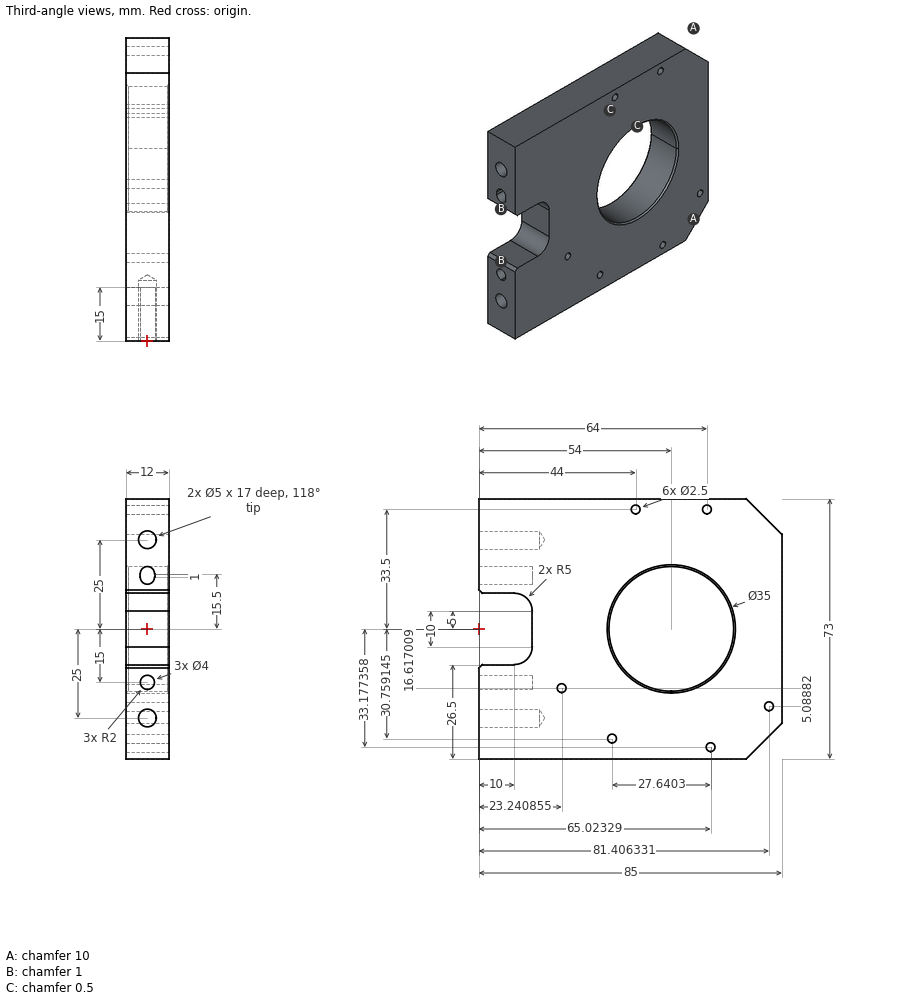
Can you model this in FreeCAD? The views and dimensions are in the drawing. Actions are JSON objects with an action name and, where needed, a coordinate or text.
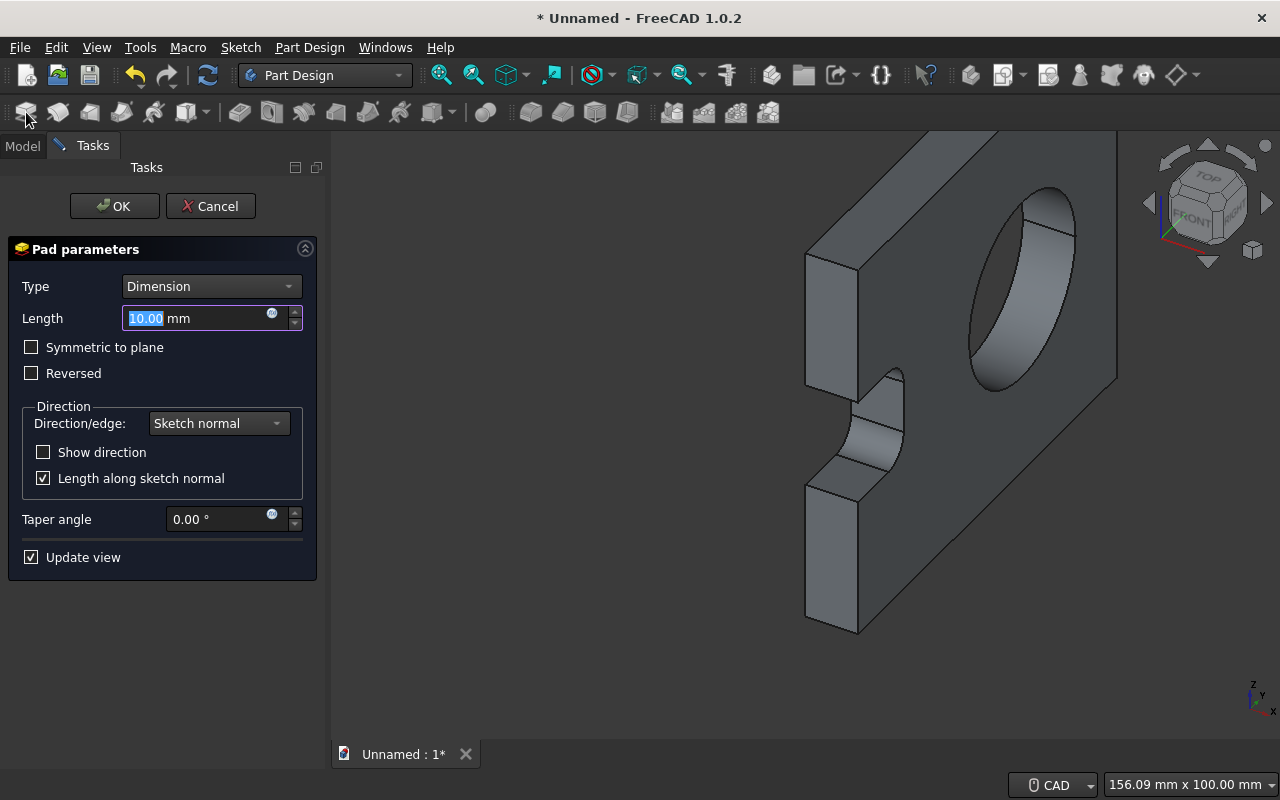
{"action": "type", "text": "12"}
{"action": "key", "text": "Tab"}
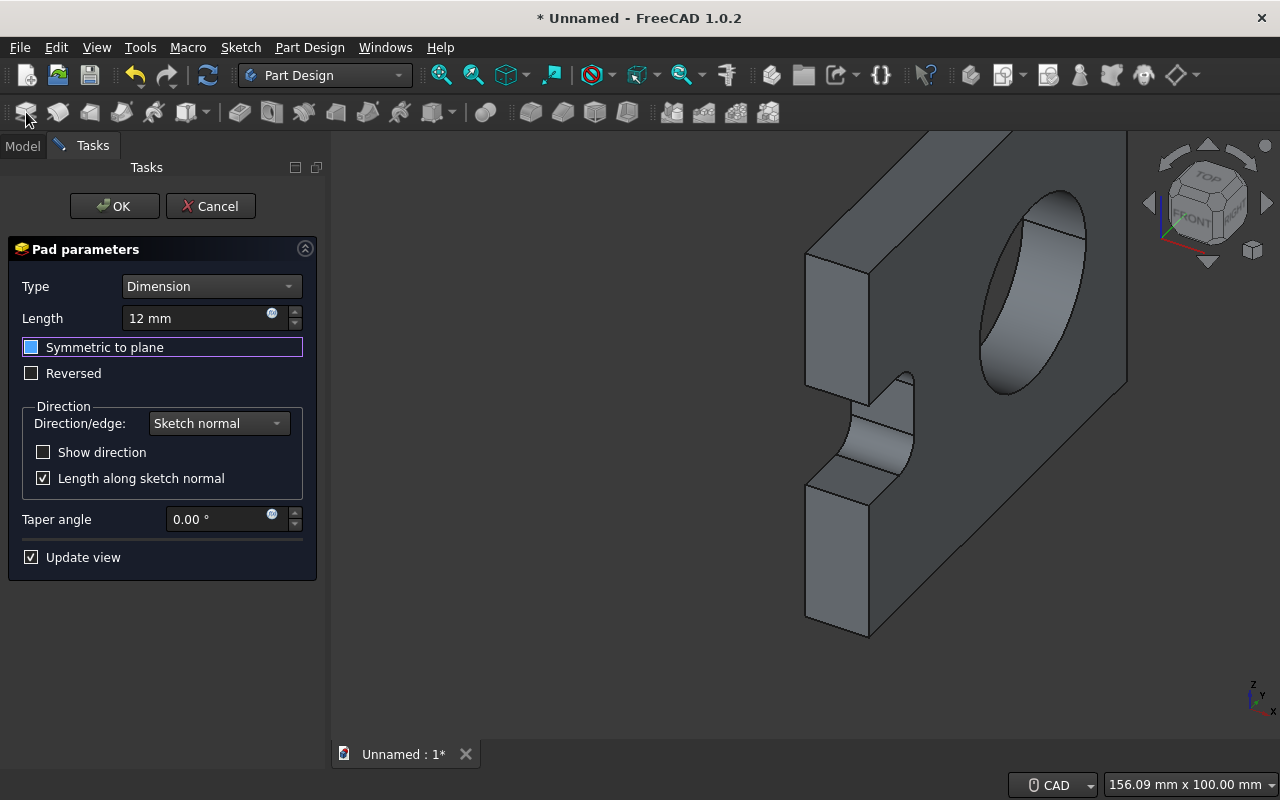
{"action": "left_click", "coordinate": [30, 347]}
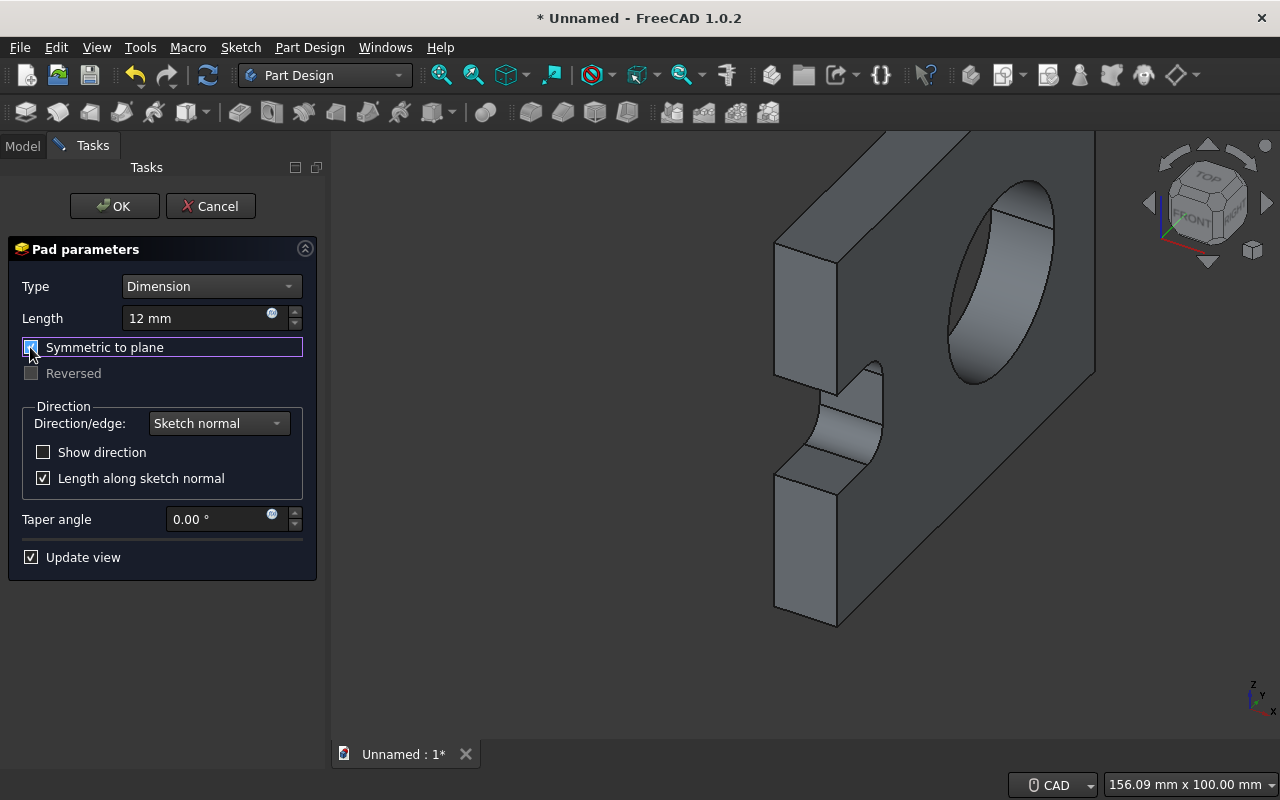
{"action": "left_click", "coordinate": [115, 206]}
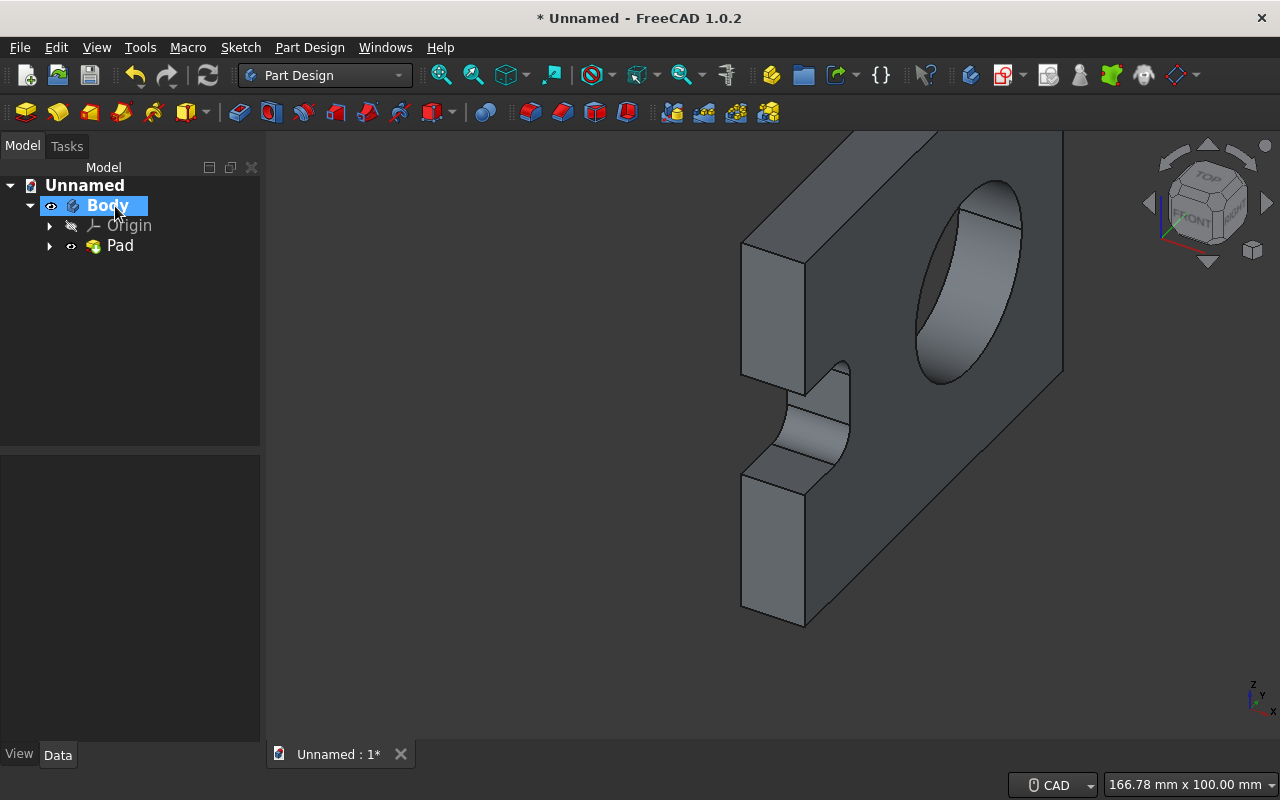
{"action": "left_click", "coordinate": [442, 76]}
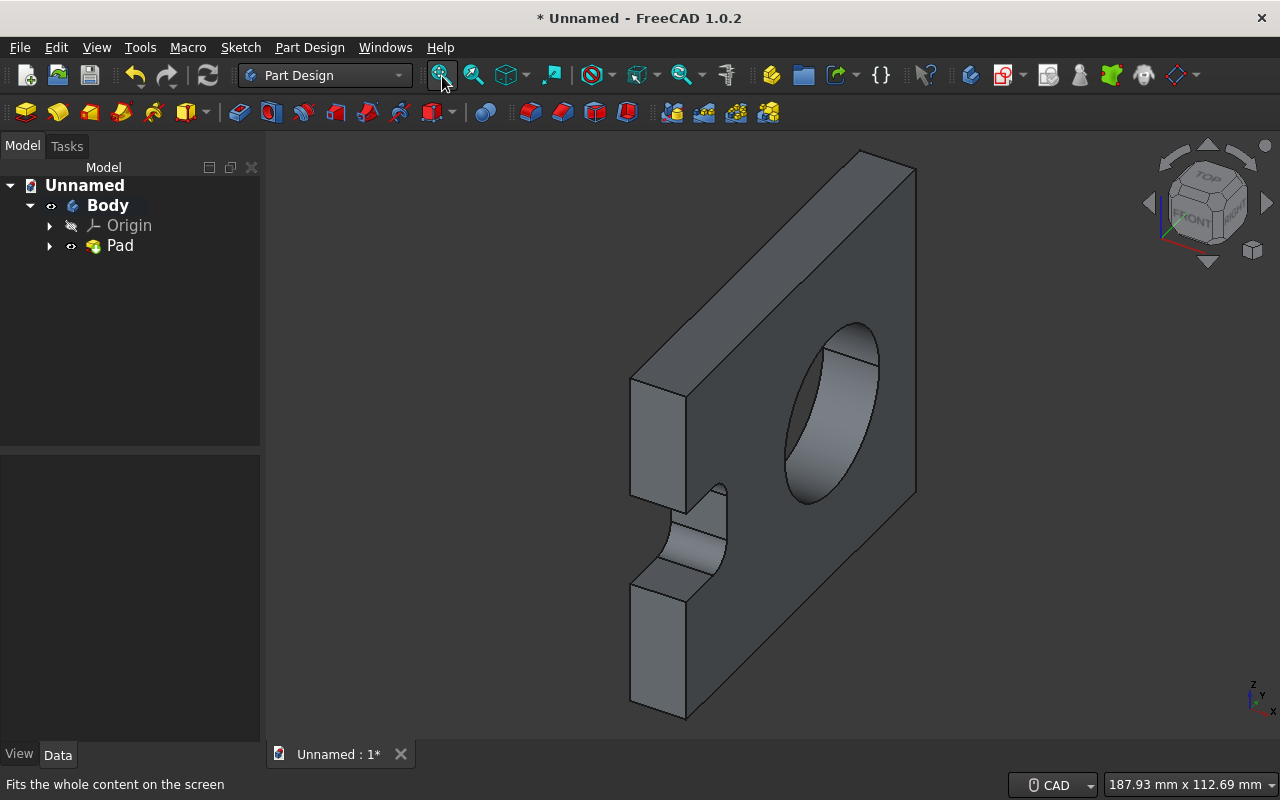
{"action": "key", "text": "0"}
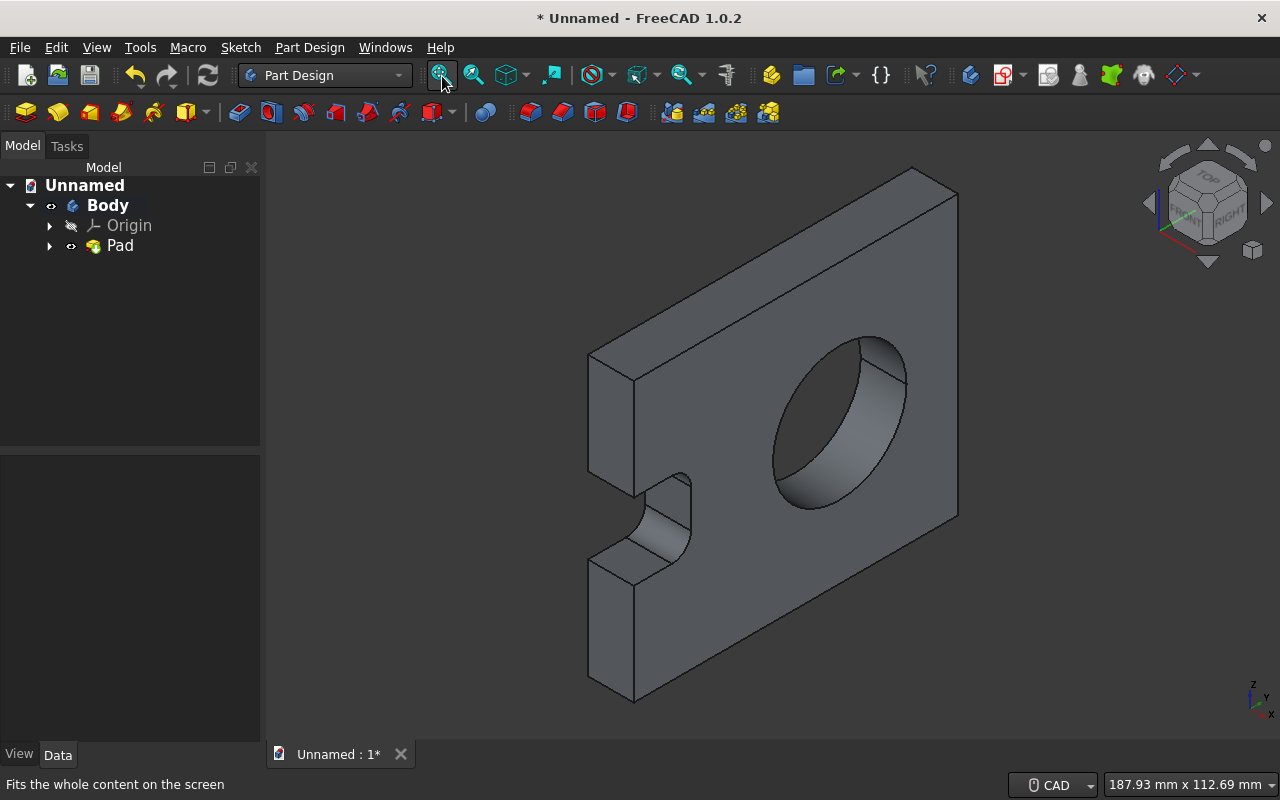
{"action": "key", "text": "2"}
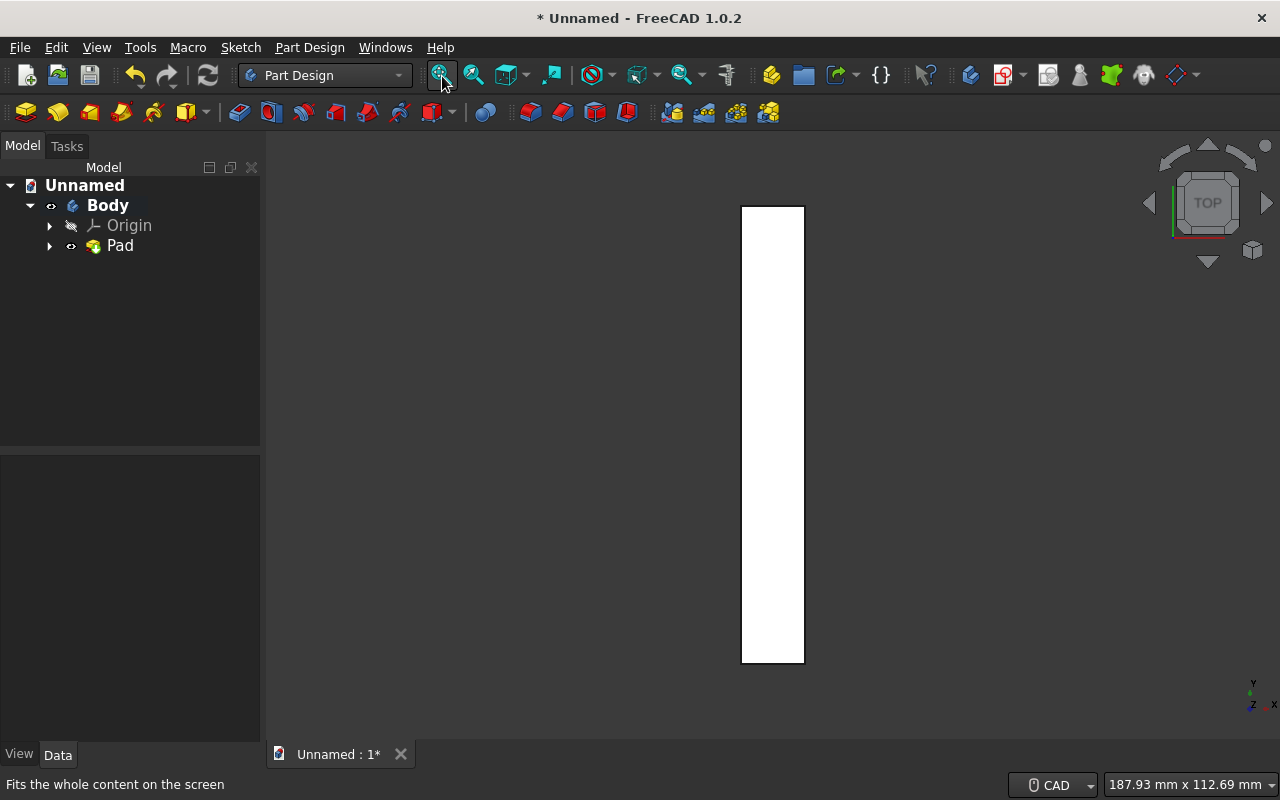
{"action": "left_click", "coordinate": [773, 205]}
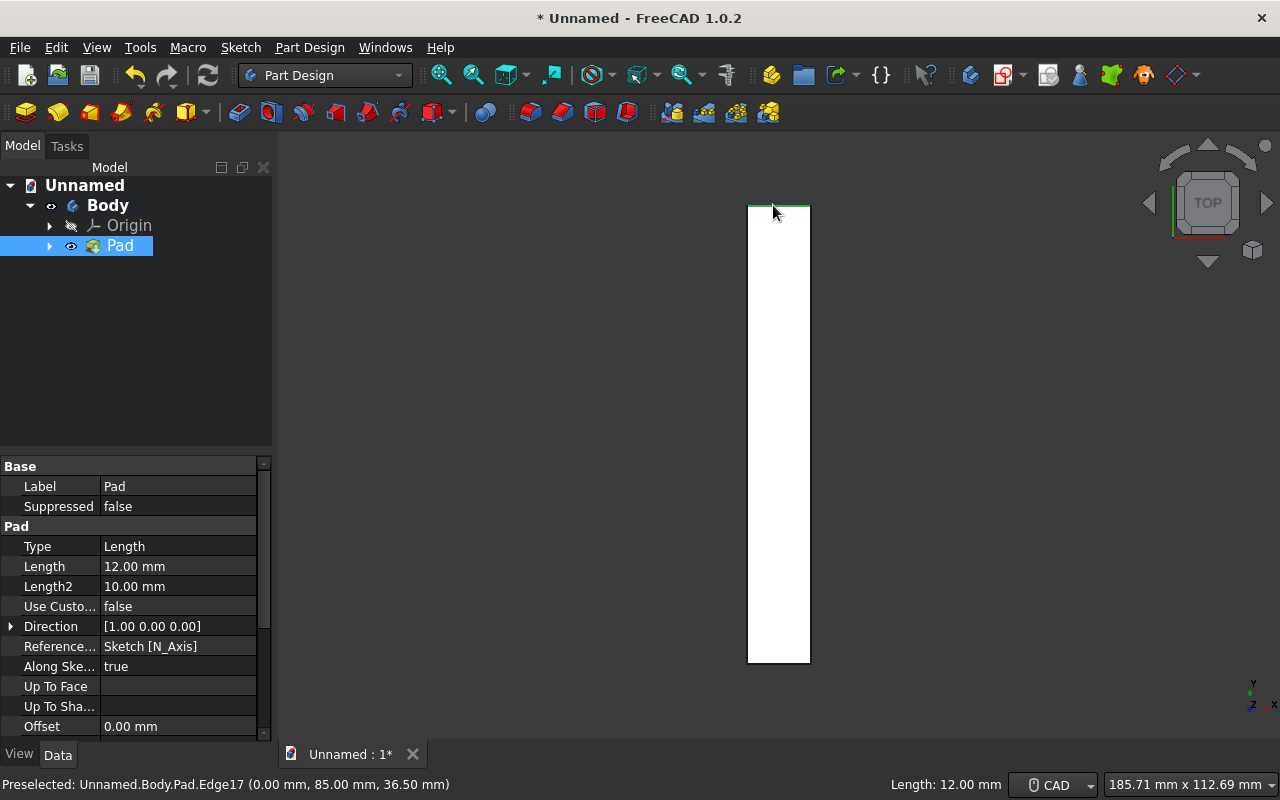
{"action": "key", "text": "1"}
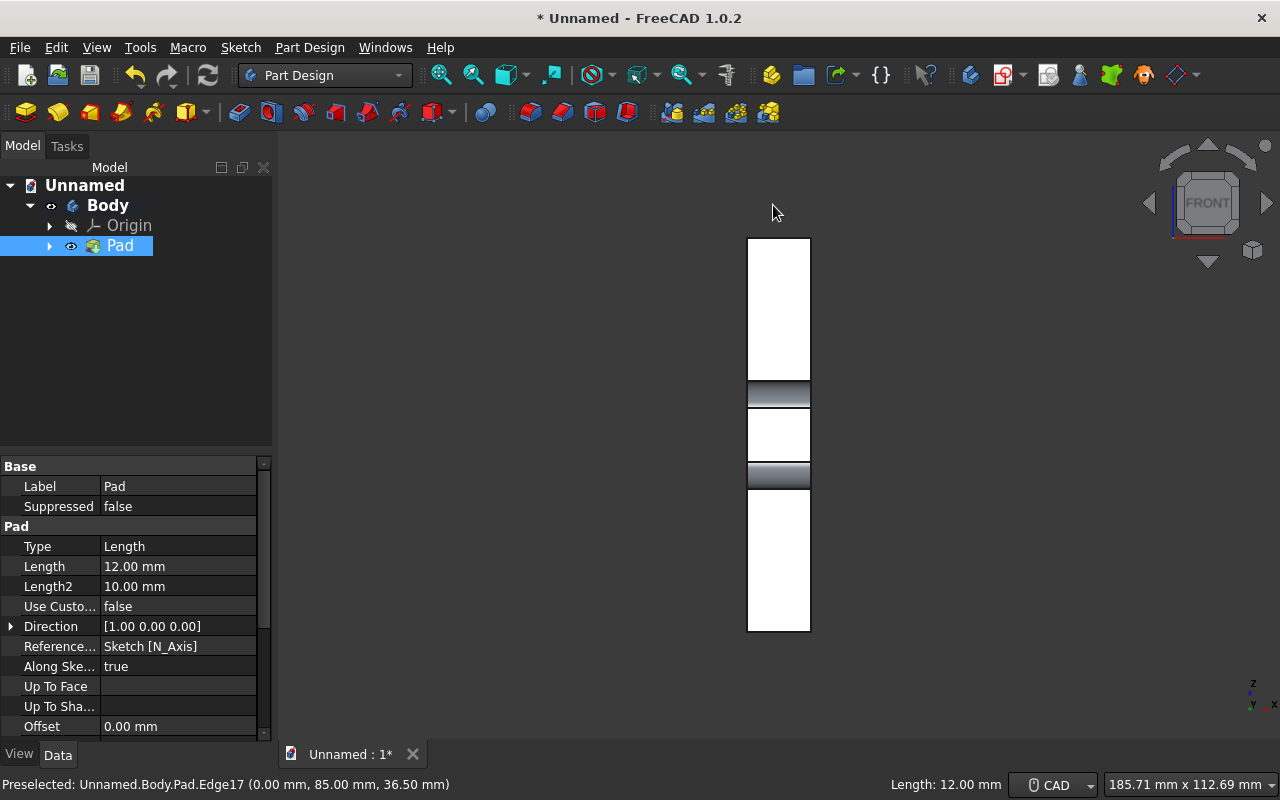
{"action": "key", "text": "3"}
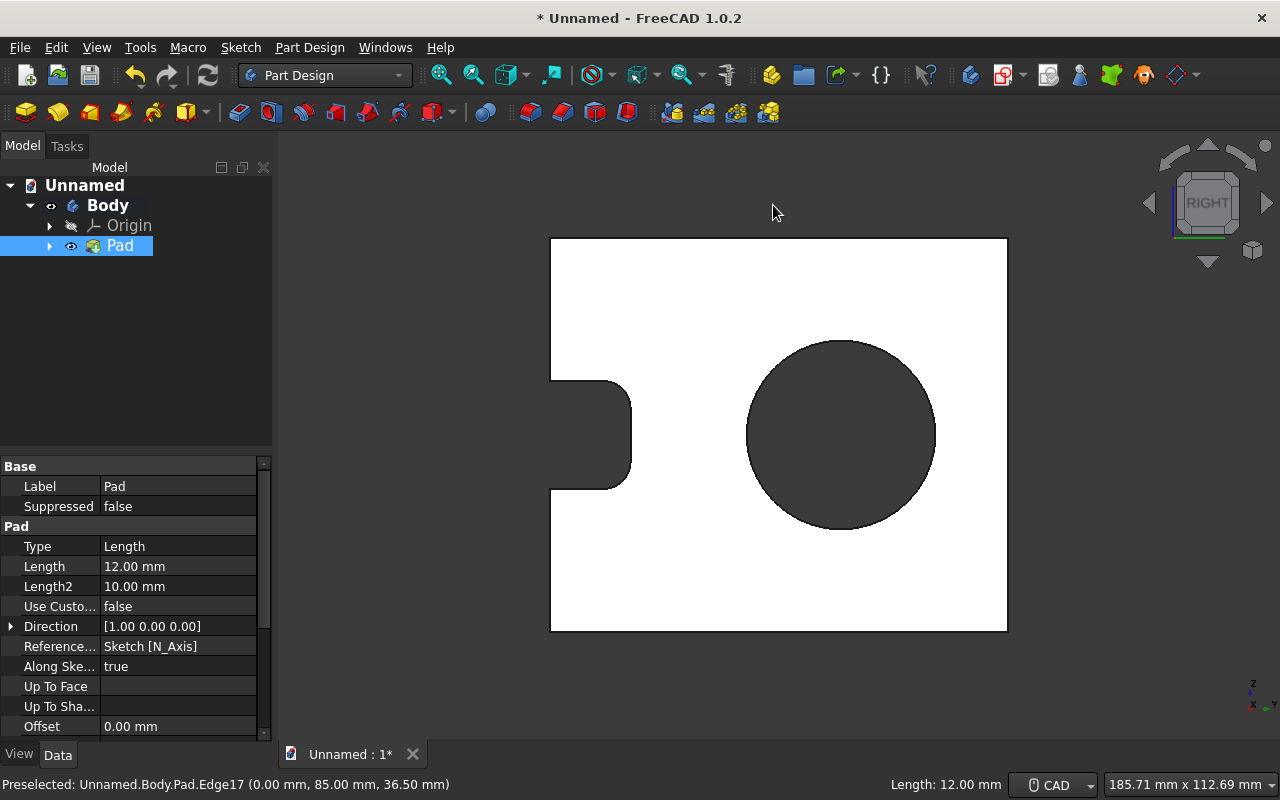
{"action": "key", "text": "5"}